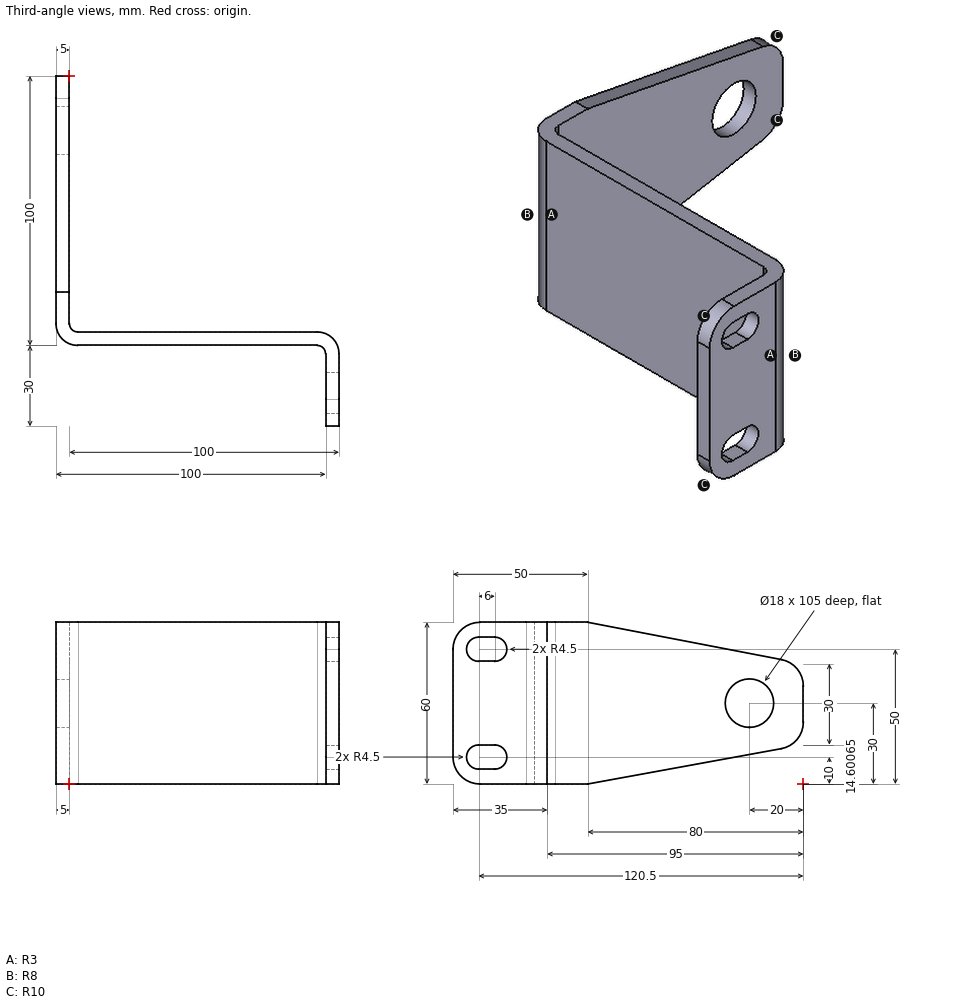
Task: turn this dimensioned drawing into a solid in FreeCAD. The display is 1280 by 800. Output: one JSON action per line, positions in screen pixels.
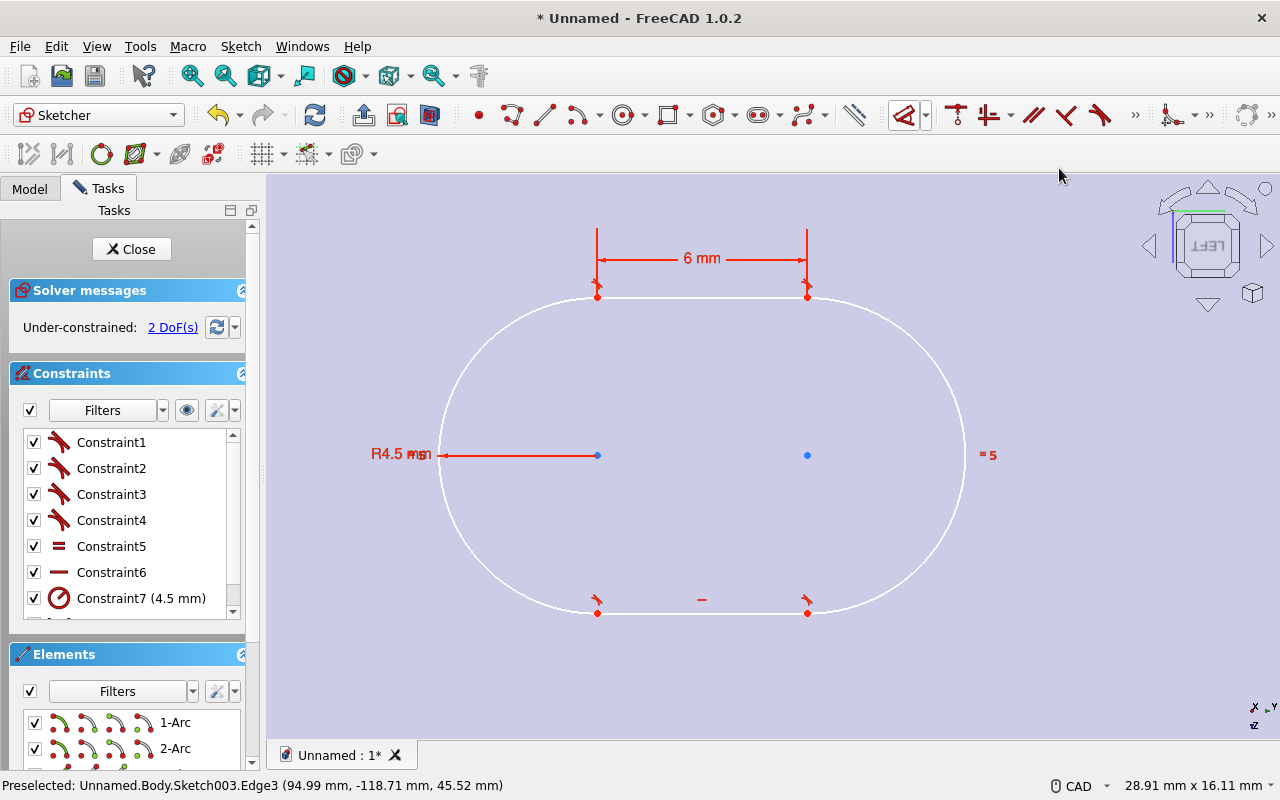
{"action": "left_click", "coordinate": [597, 456]}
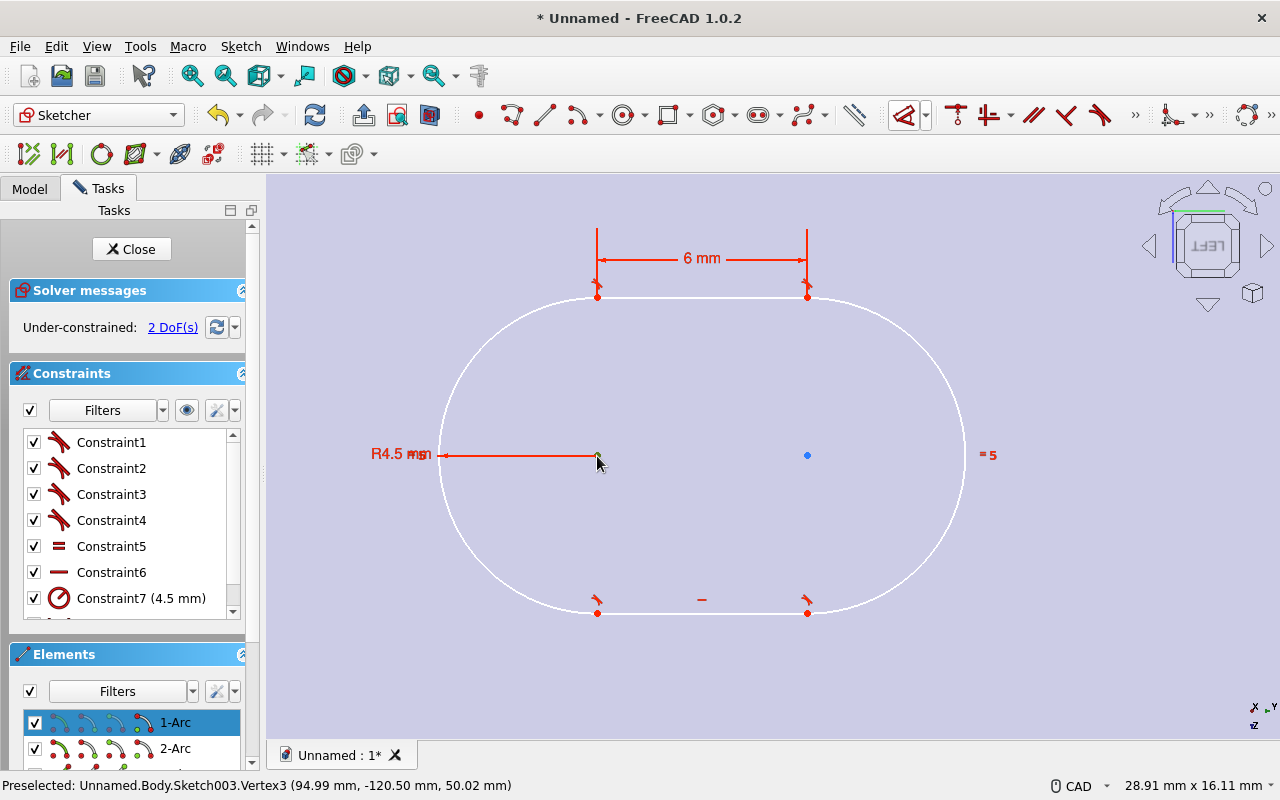
{"action": "left_click", "coordinate": [926, 116]}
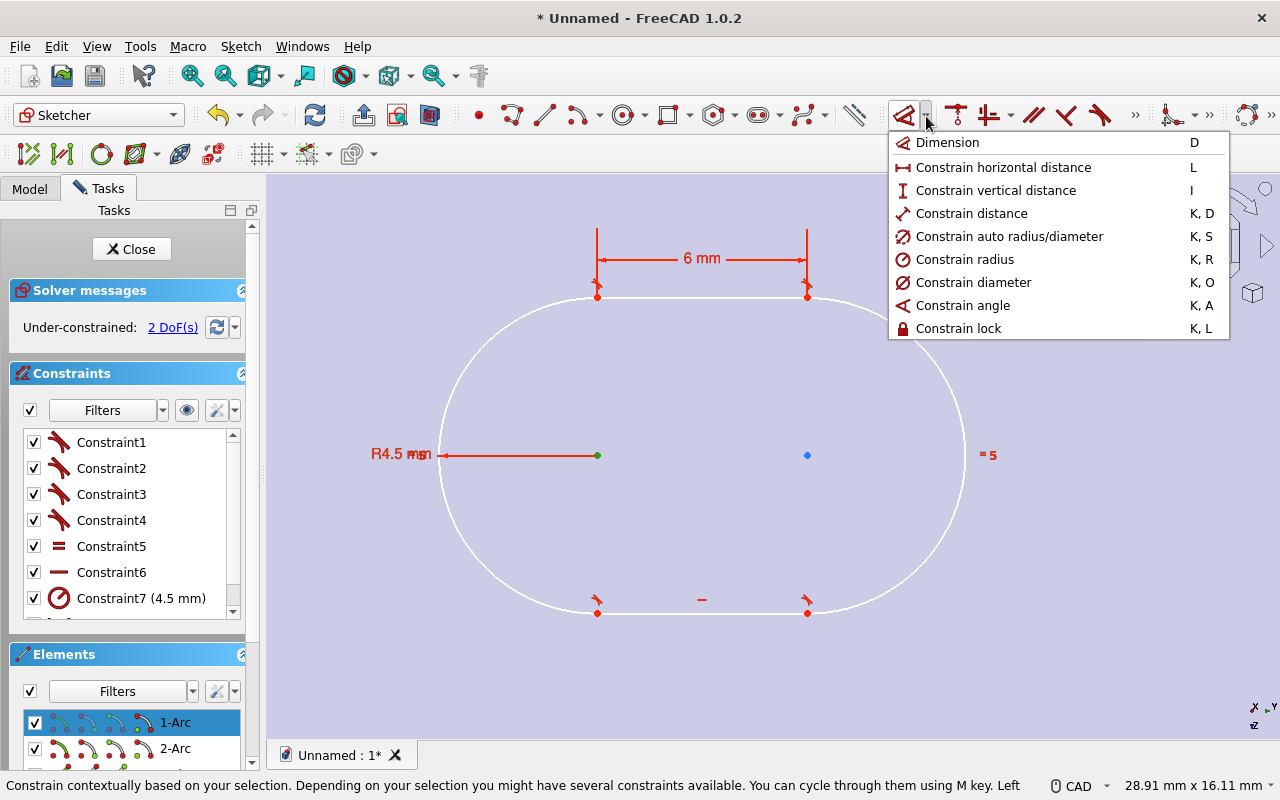
{"action": "left_click", "coordinate": [1059, 190]}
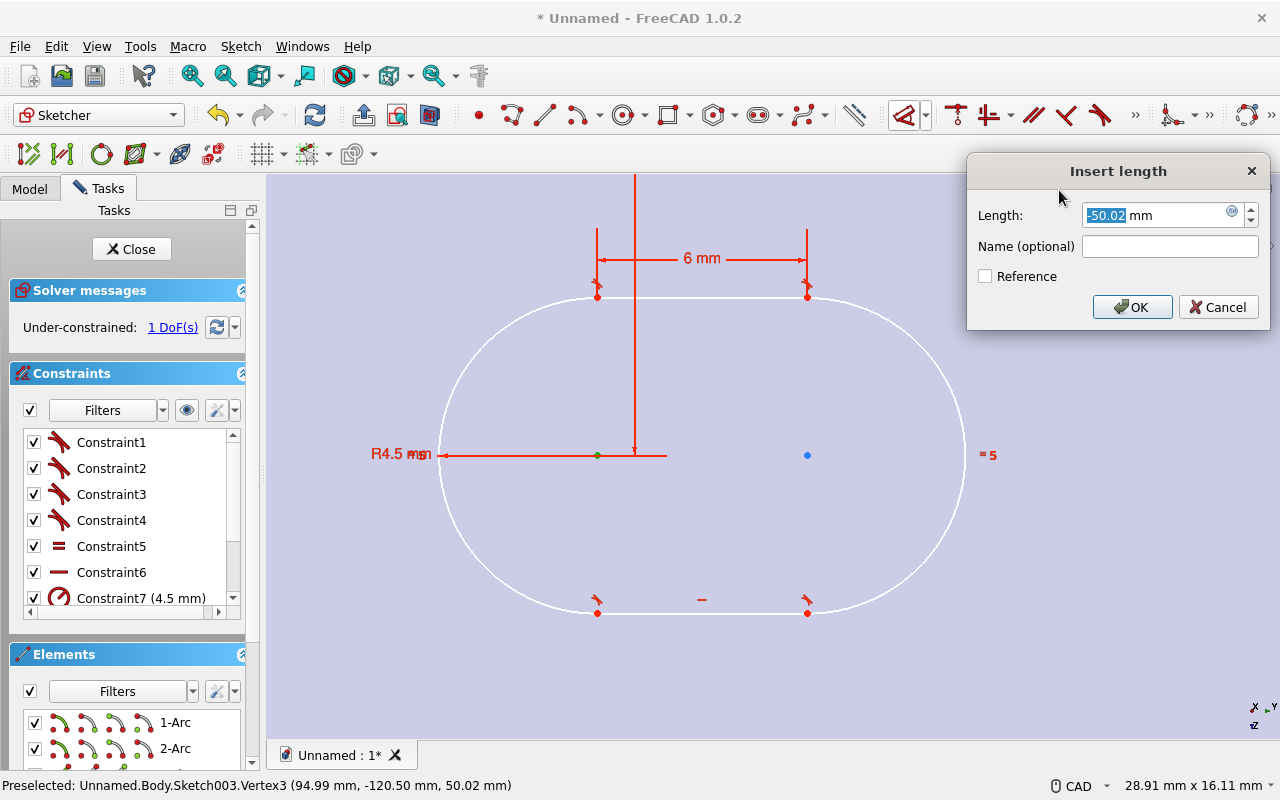
{"action": "type", "text": "-50"}
{"action": "key", "text": "Return"}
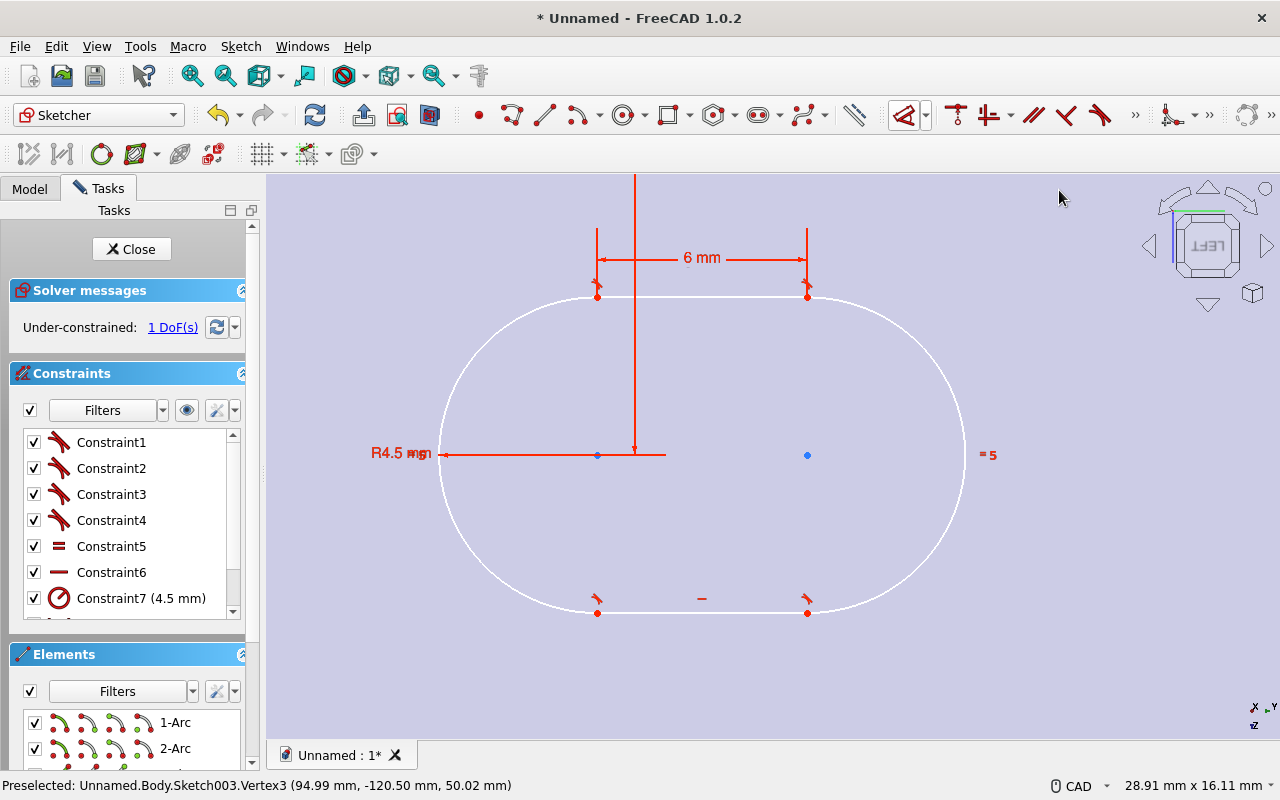
{"action": "left_click", "coordinate": [597, 297]}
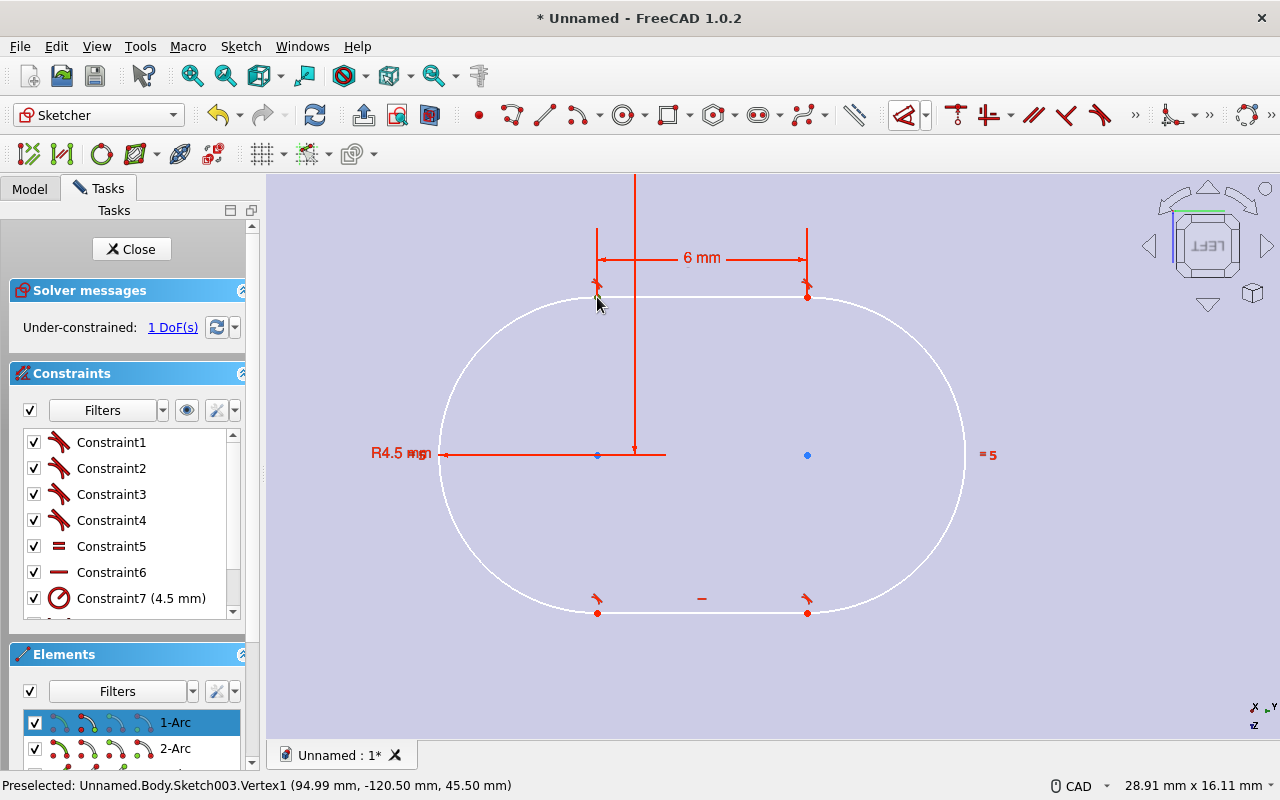
{"action": "key", "text": "l"}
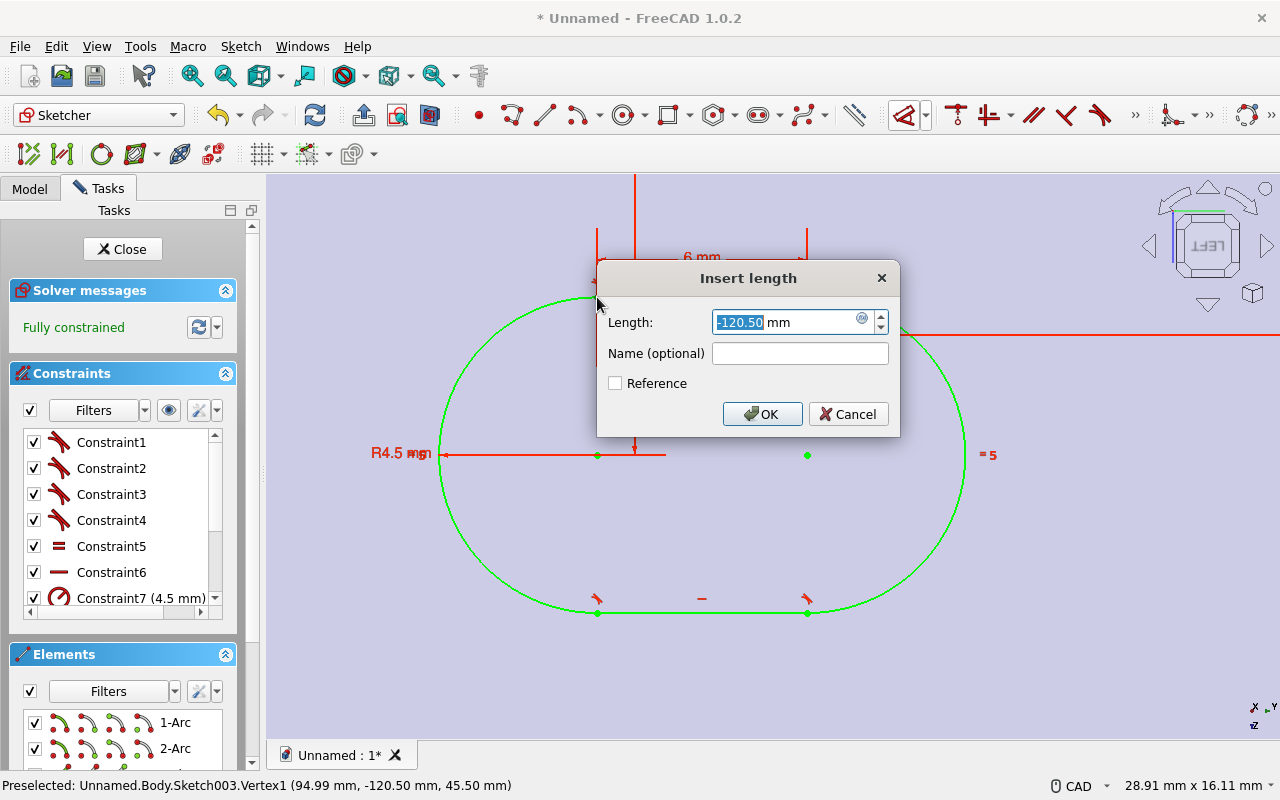
{"action": "type", "text": "-120.5"}
{"action": "key", "text": "Return"}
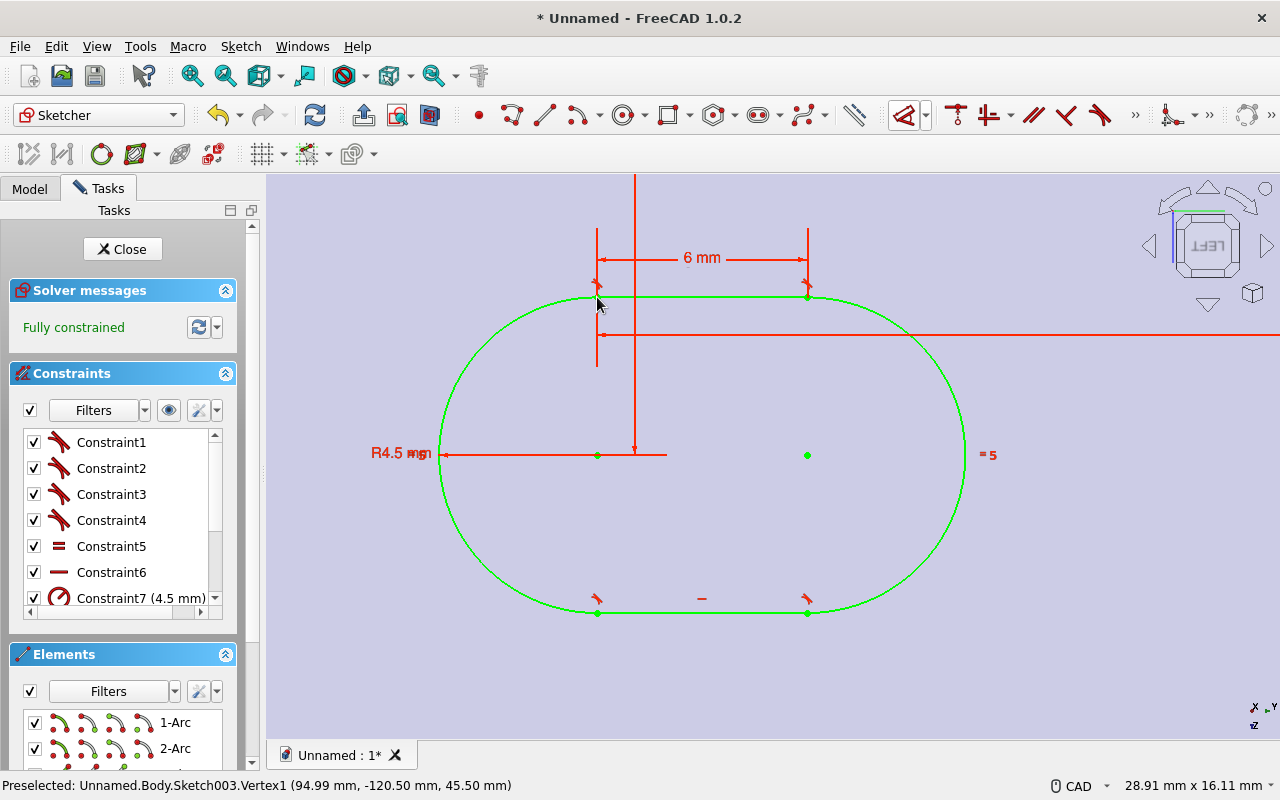
{"action": "left_click", "coordinate": [123, 249]}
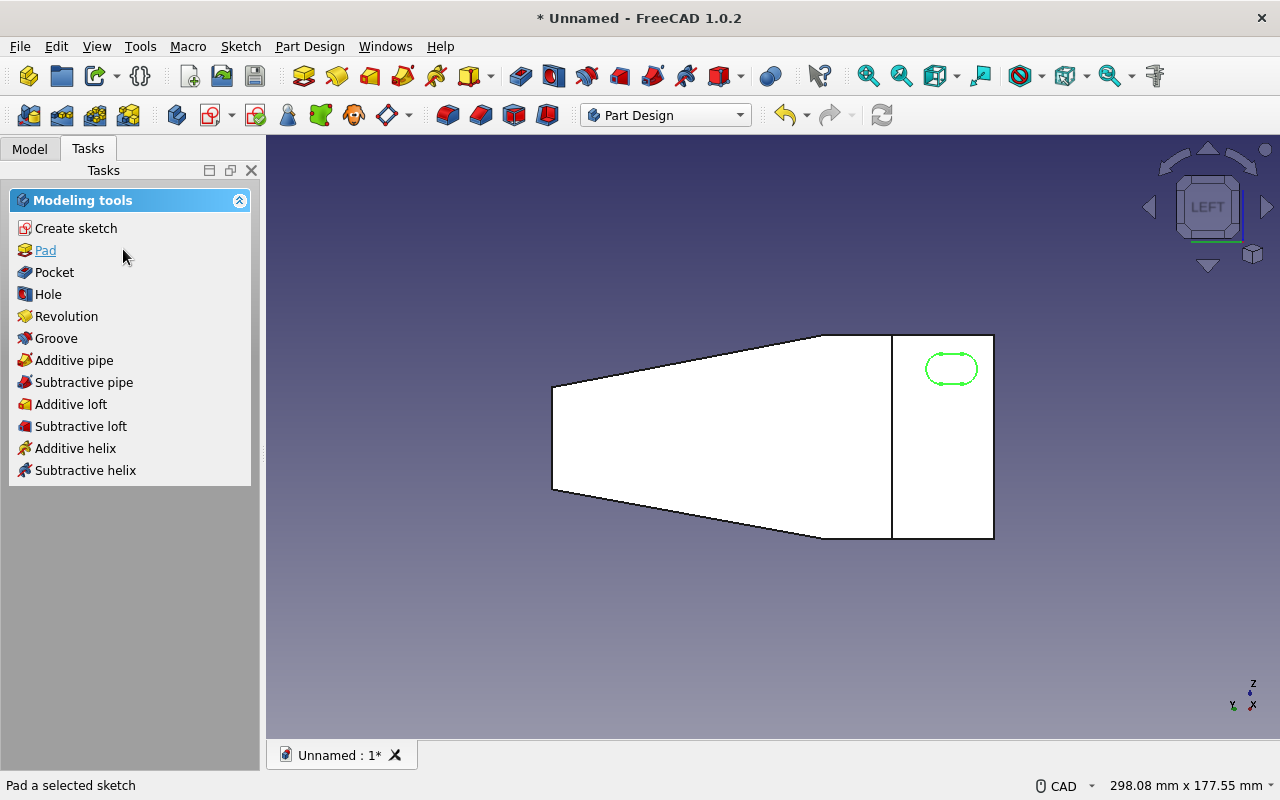
{"action": "left_click", "coordinate": [521, 76]}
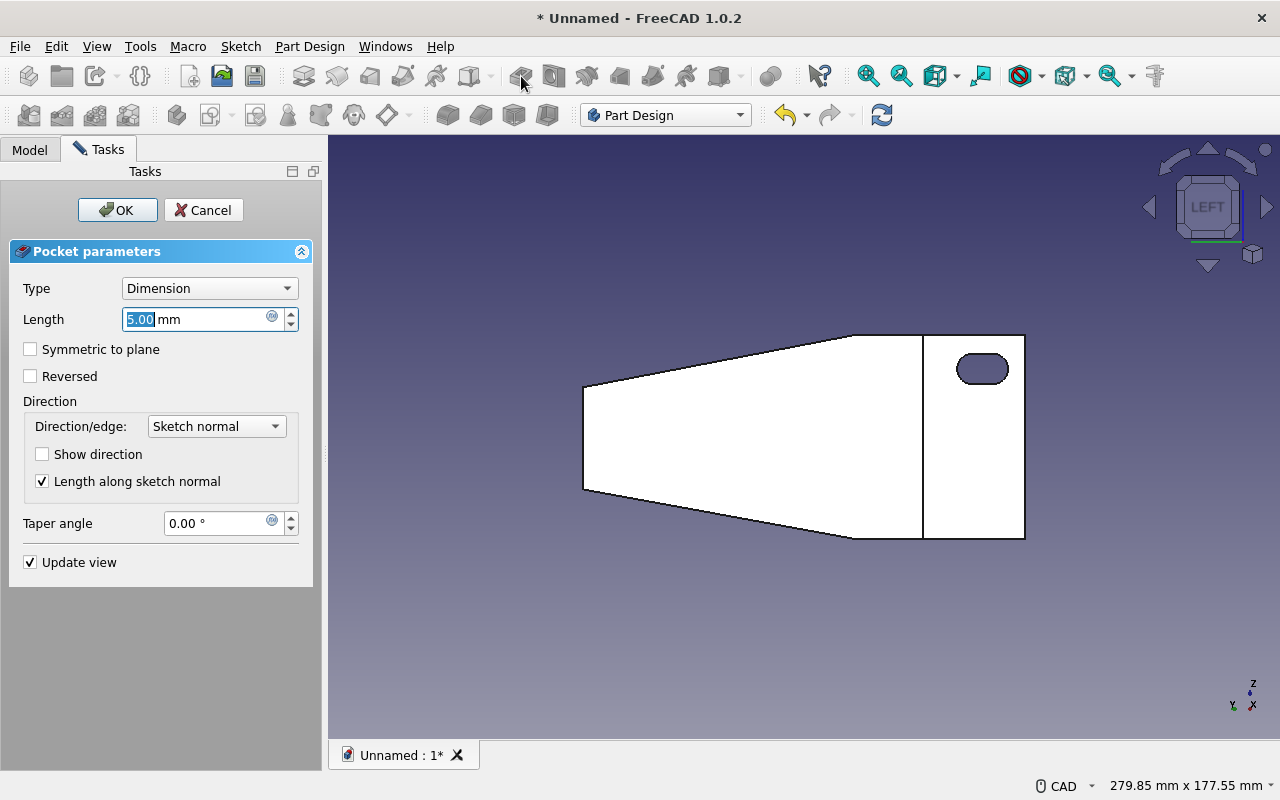
{"action": "left_click", "coordinate": [210, 288]}